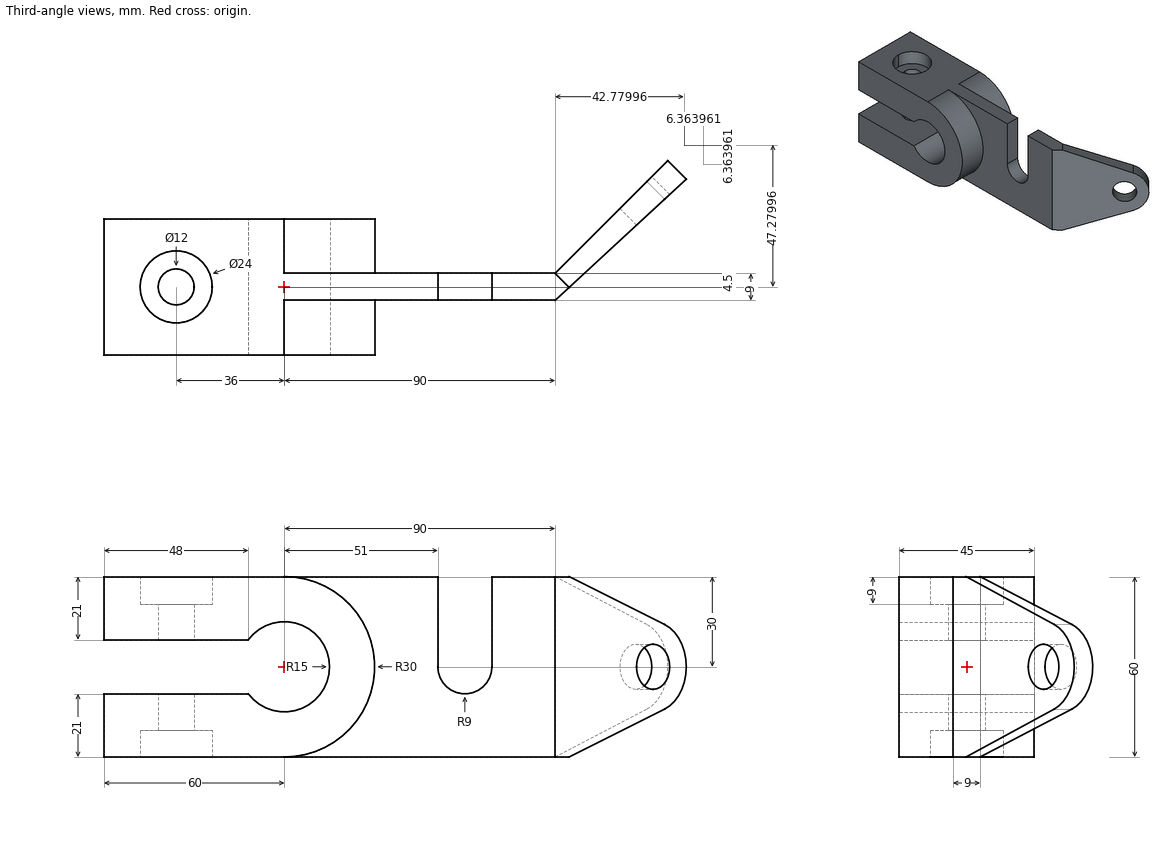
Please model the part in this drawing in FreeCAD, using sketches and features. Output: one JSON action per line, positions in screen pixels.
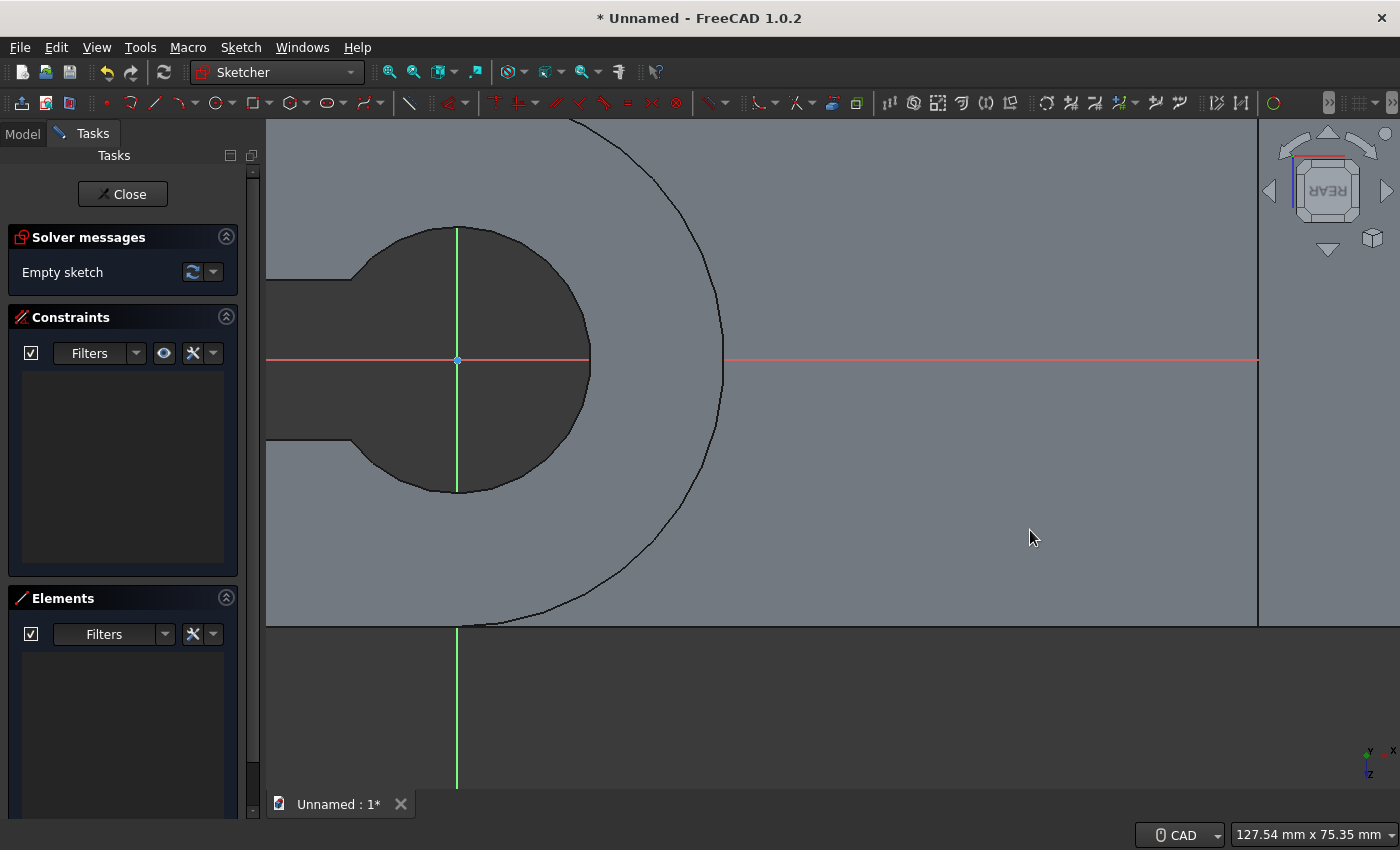
{"action": "key", "text": "g m"}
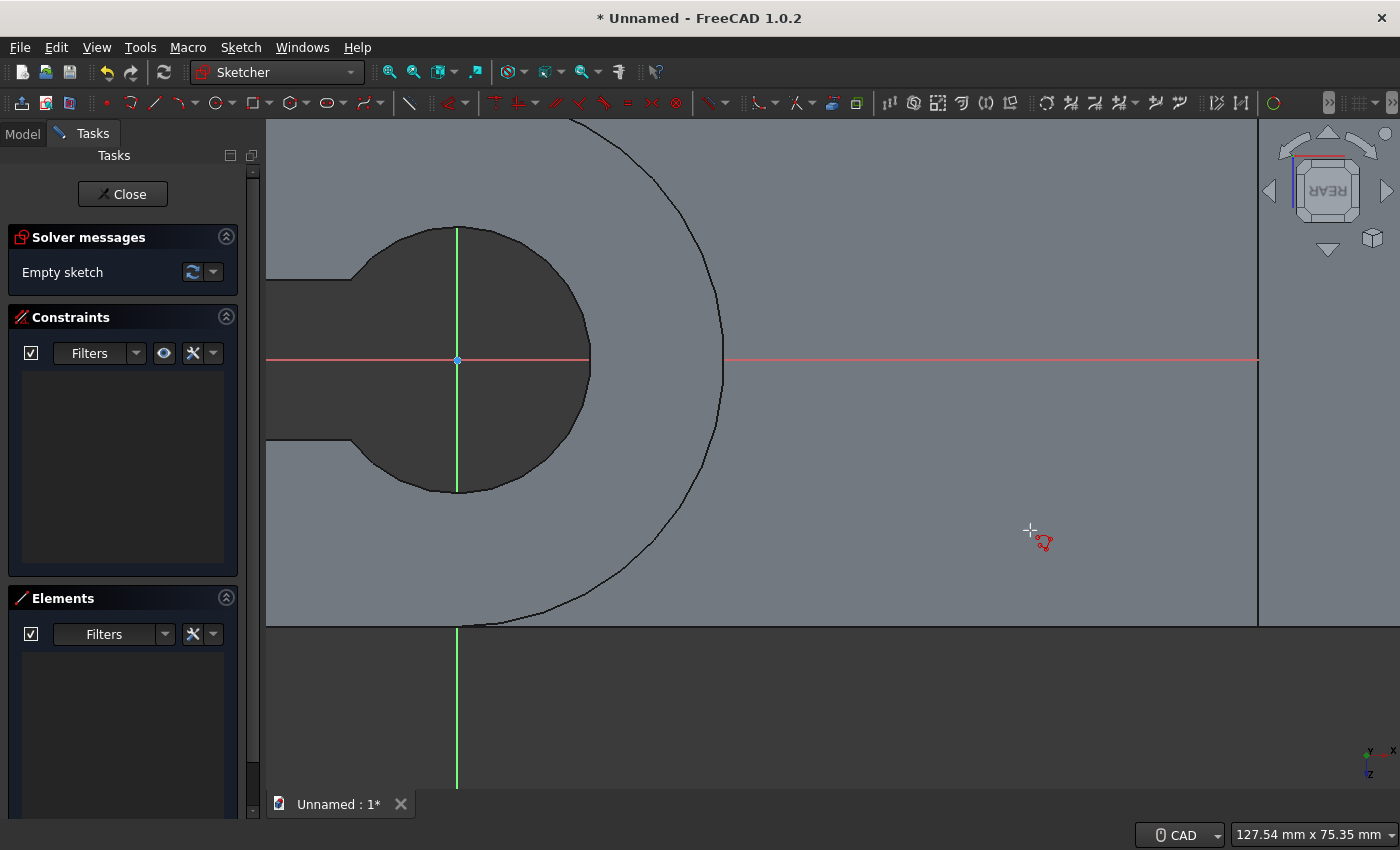
{"action": "left_click", "coordinate": [911, 360]}
{"action": "left_click", "coordinate": [911, 627]}
{"action": "left_click", "coordinate": [1071, 627]}
{"action": "left_click", "coordinate": [1071, 360]}
{"action": "right_click", "coordinate": [1071, 360]}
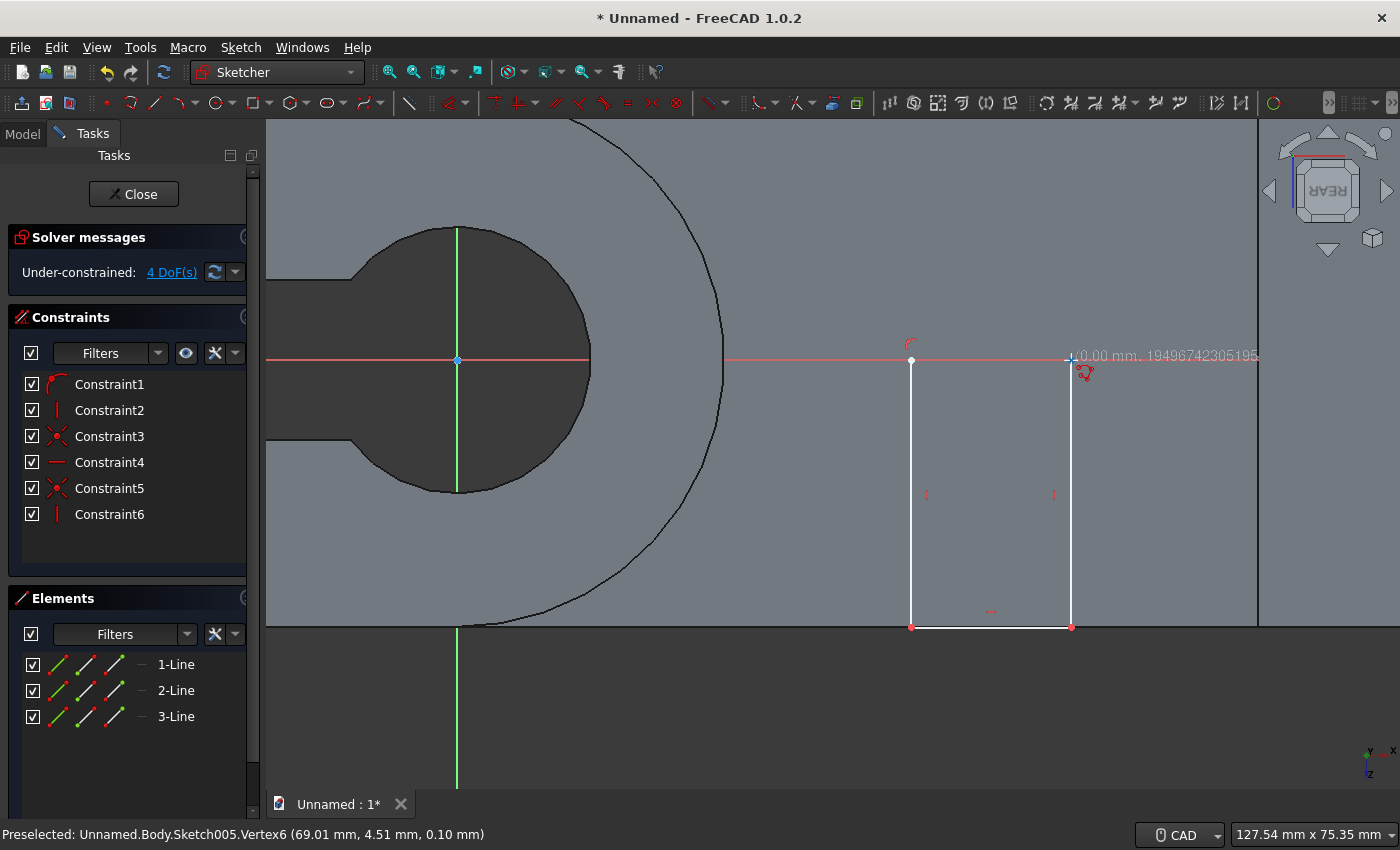
{"action": "key", "text": "g 3 a"}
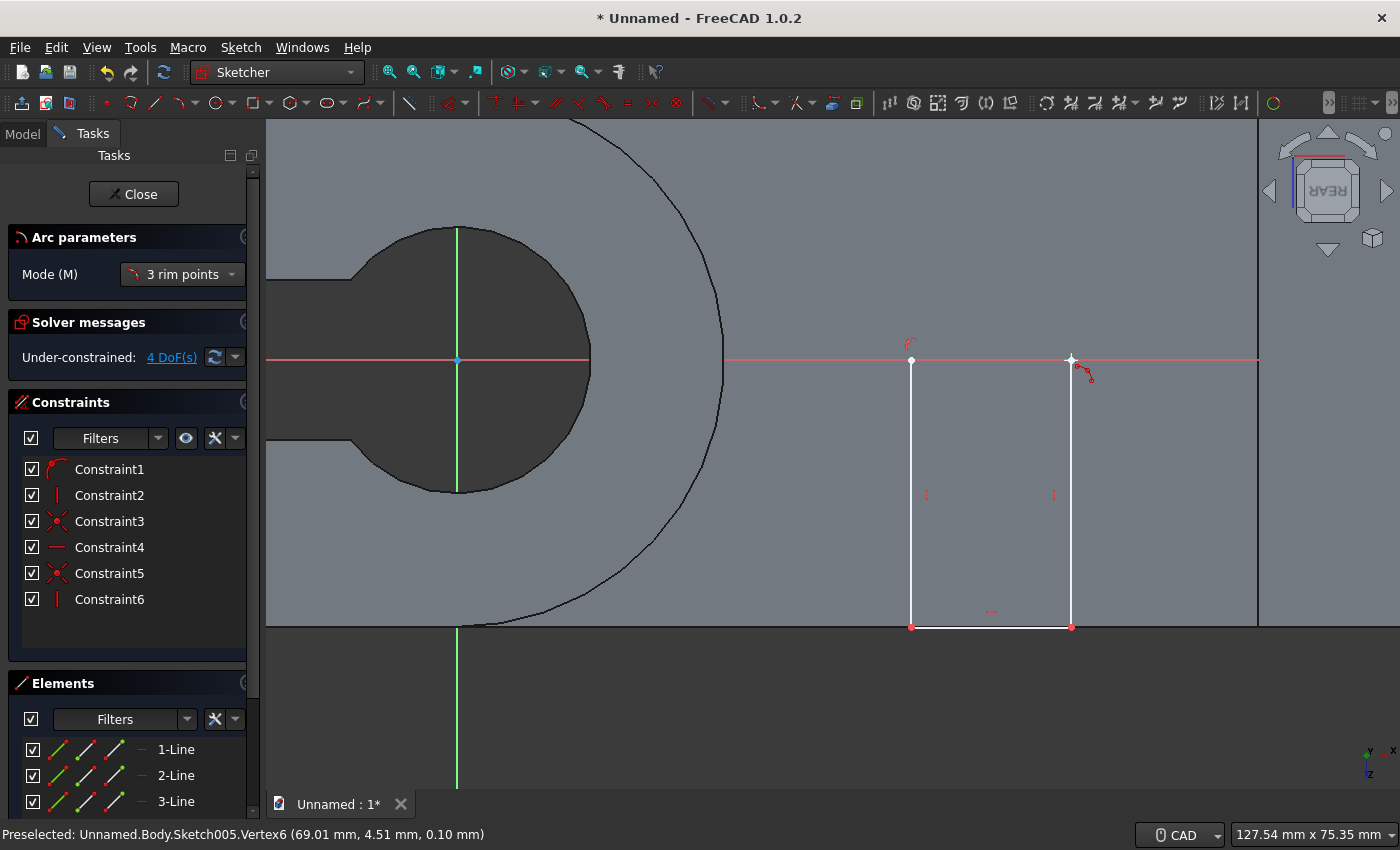
{"action": "left_click", "coordinate": [1071, 361]}
{"action": "left_click", "coordinate": [911, 360]}
{"action": "left_click", "coordinate": [991, 280]}
{"action": "key", "text": "Escape"}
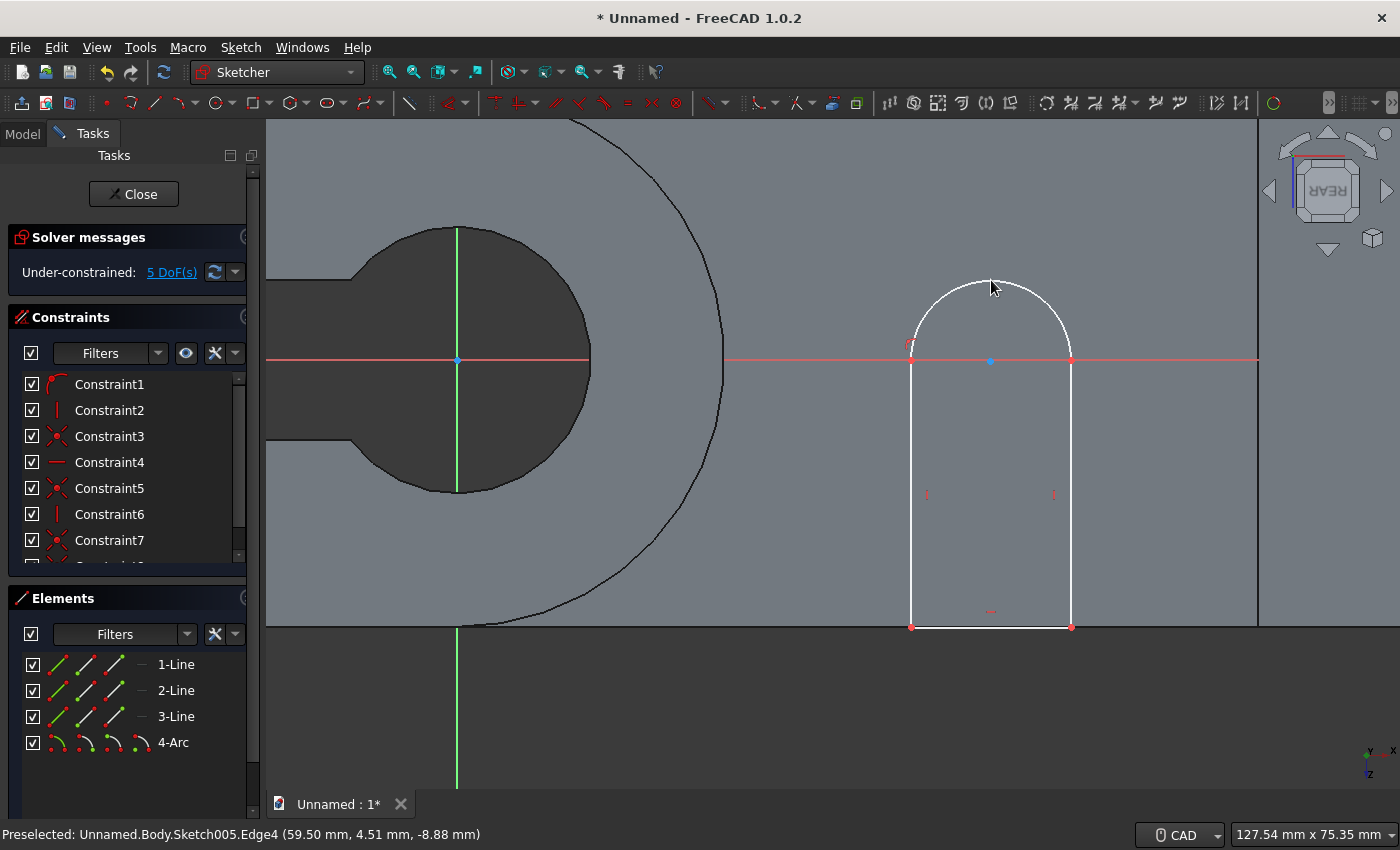
{"action": "left_click", "coordinate": [911, 440]}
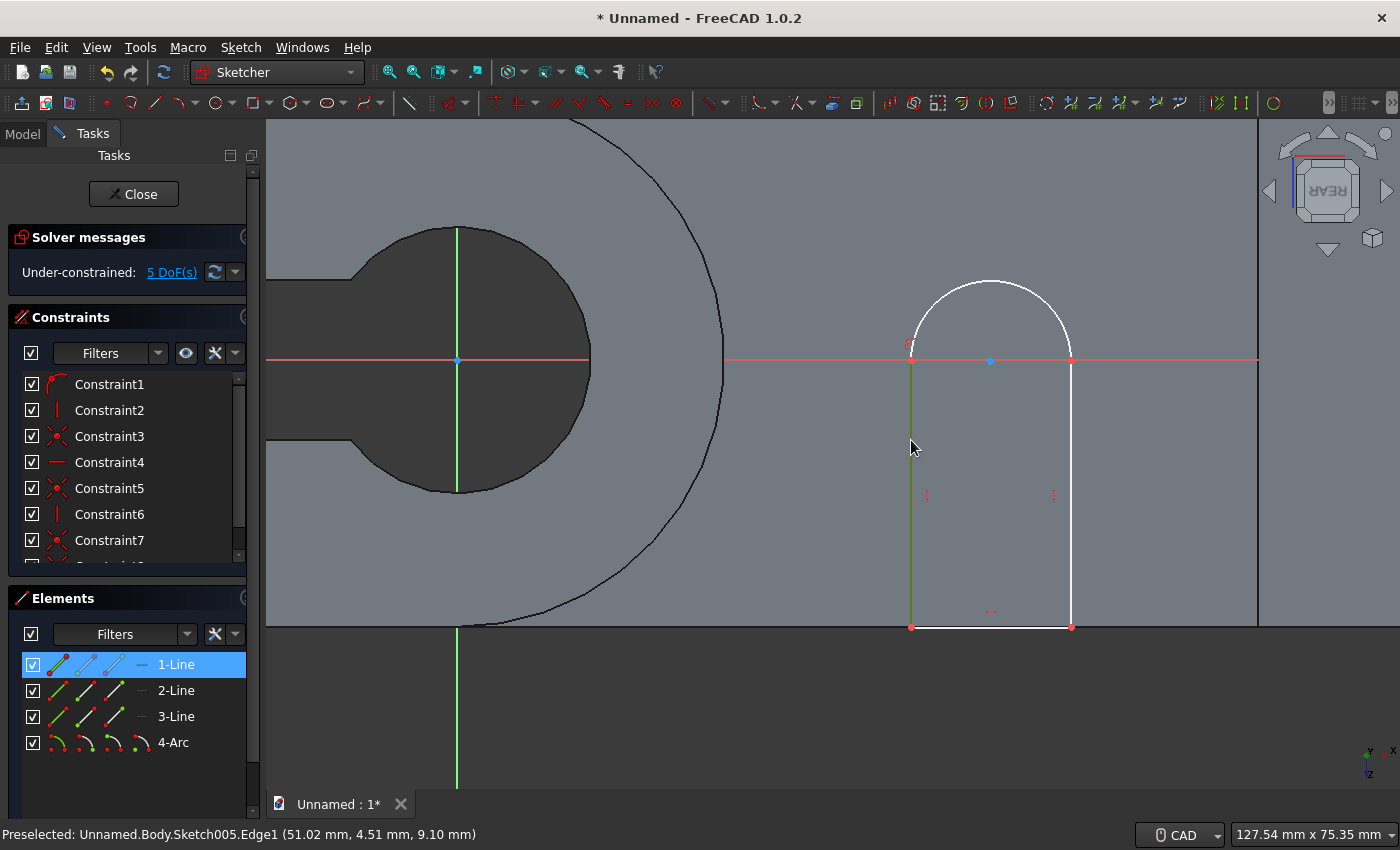
{"action": "left_click", "coordinate": [1038, 296]}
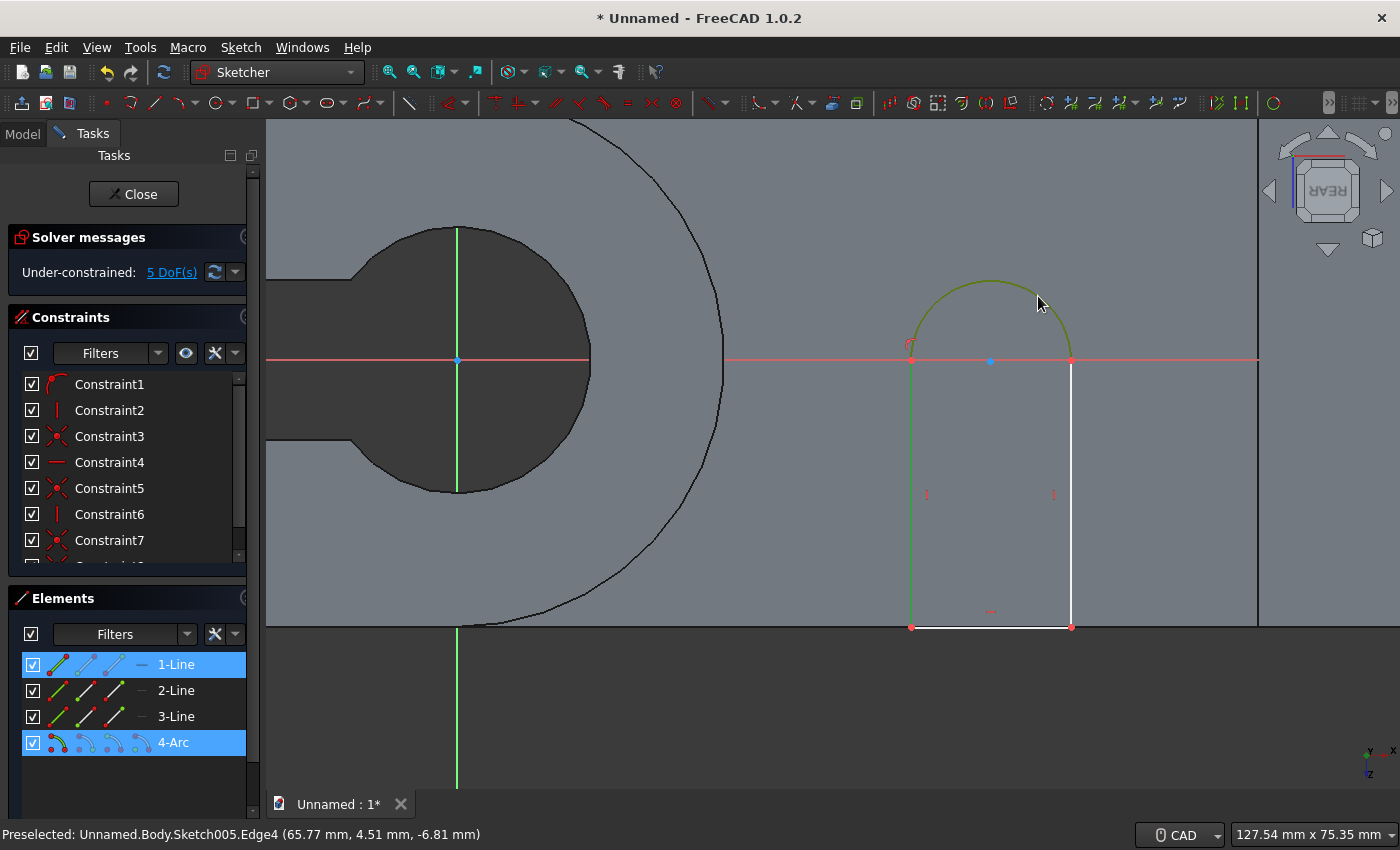
{"action": "key", "text": "t"}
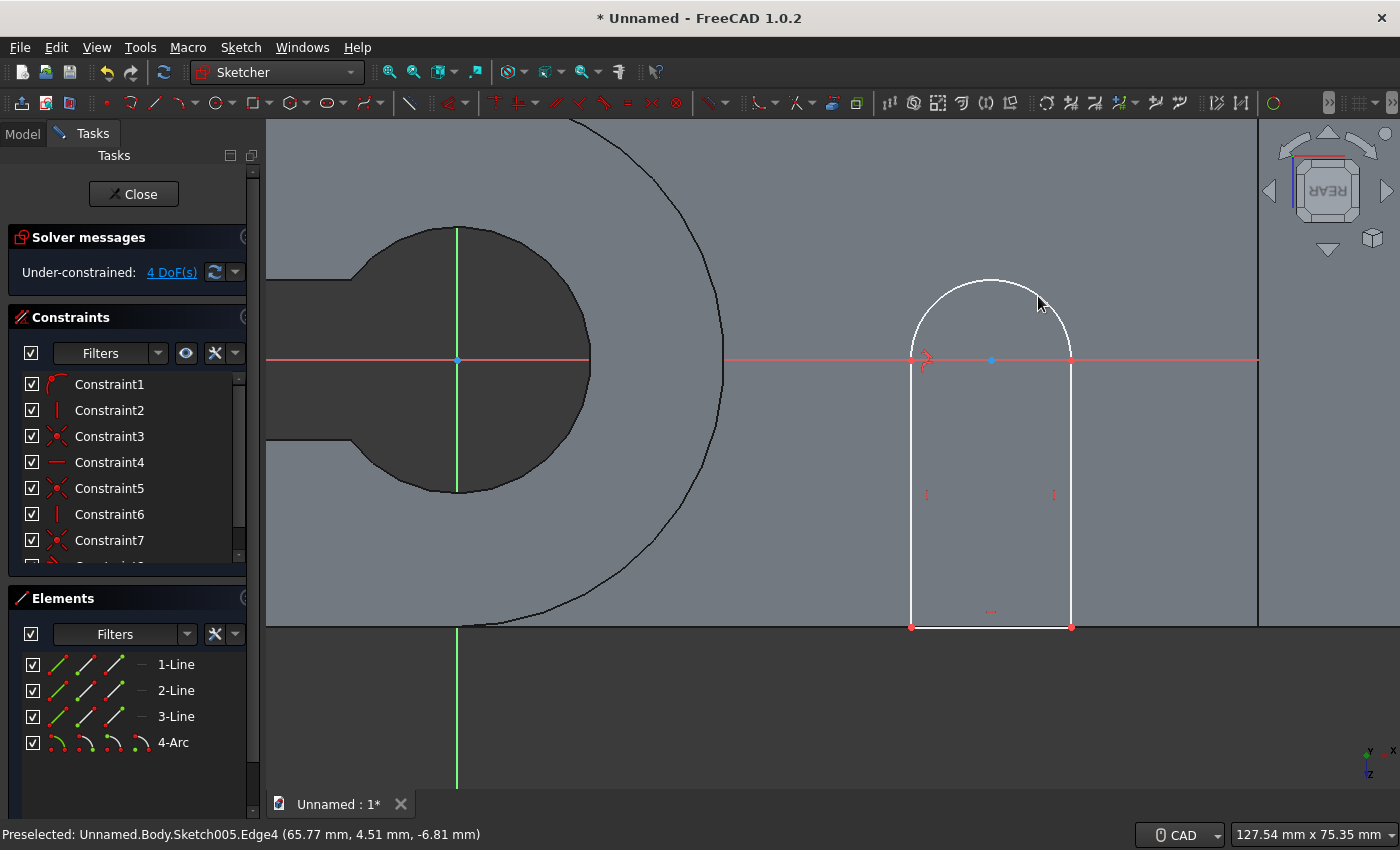
{"action": "left_click", "coordinate": [1071, 548]}